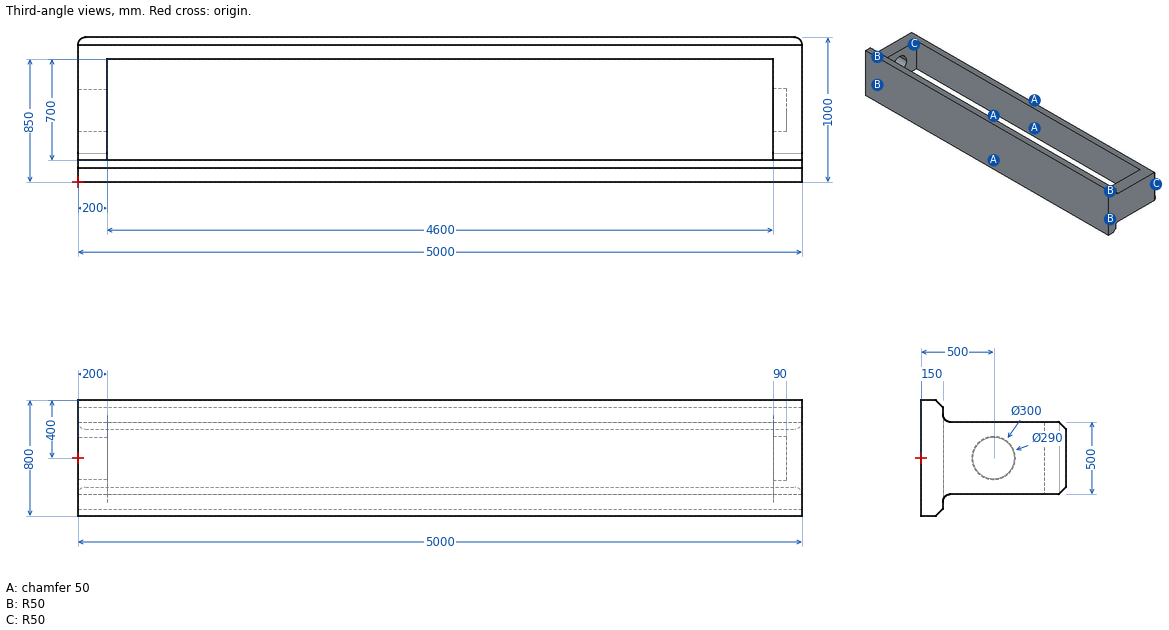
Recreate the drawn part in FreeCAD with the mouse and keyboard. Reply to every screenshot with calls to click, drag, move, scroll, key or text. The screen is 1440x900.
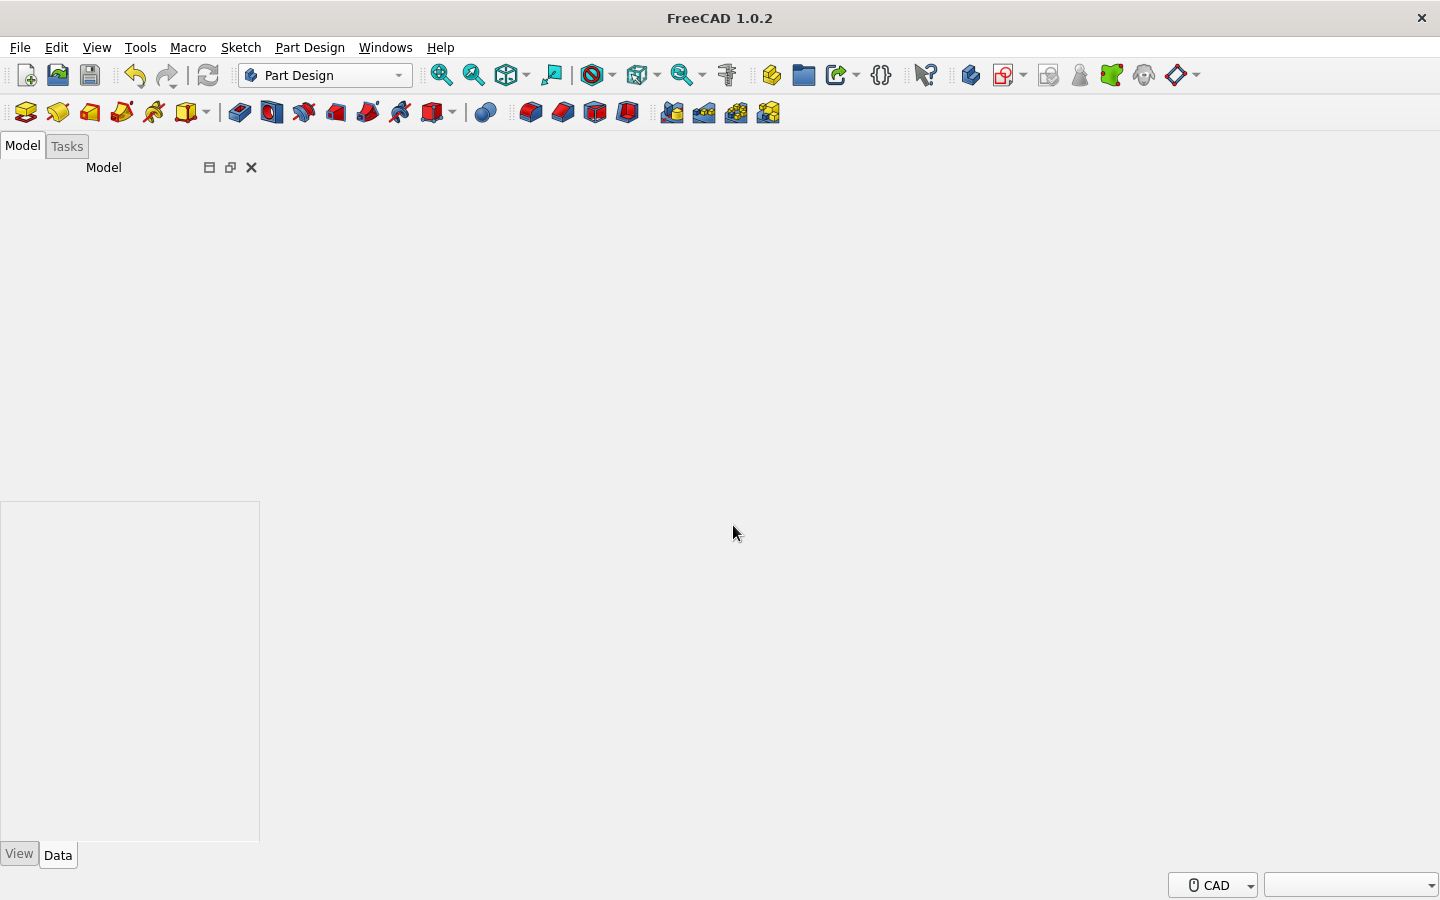
key(ctrl+n)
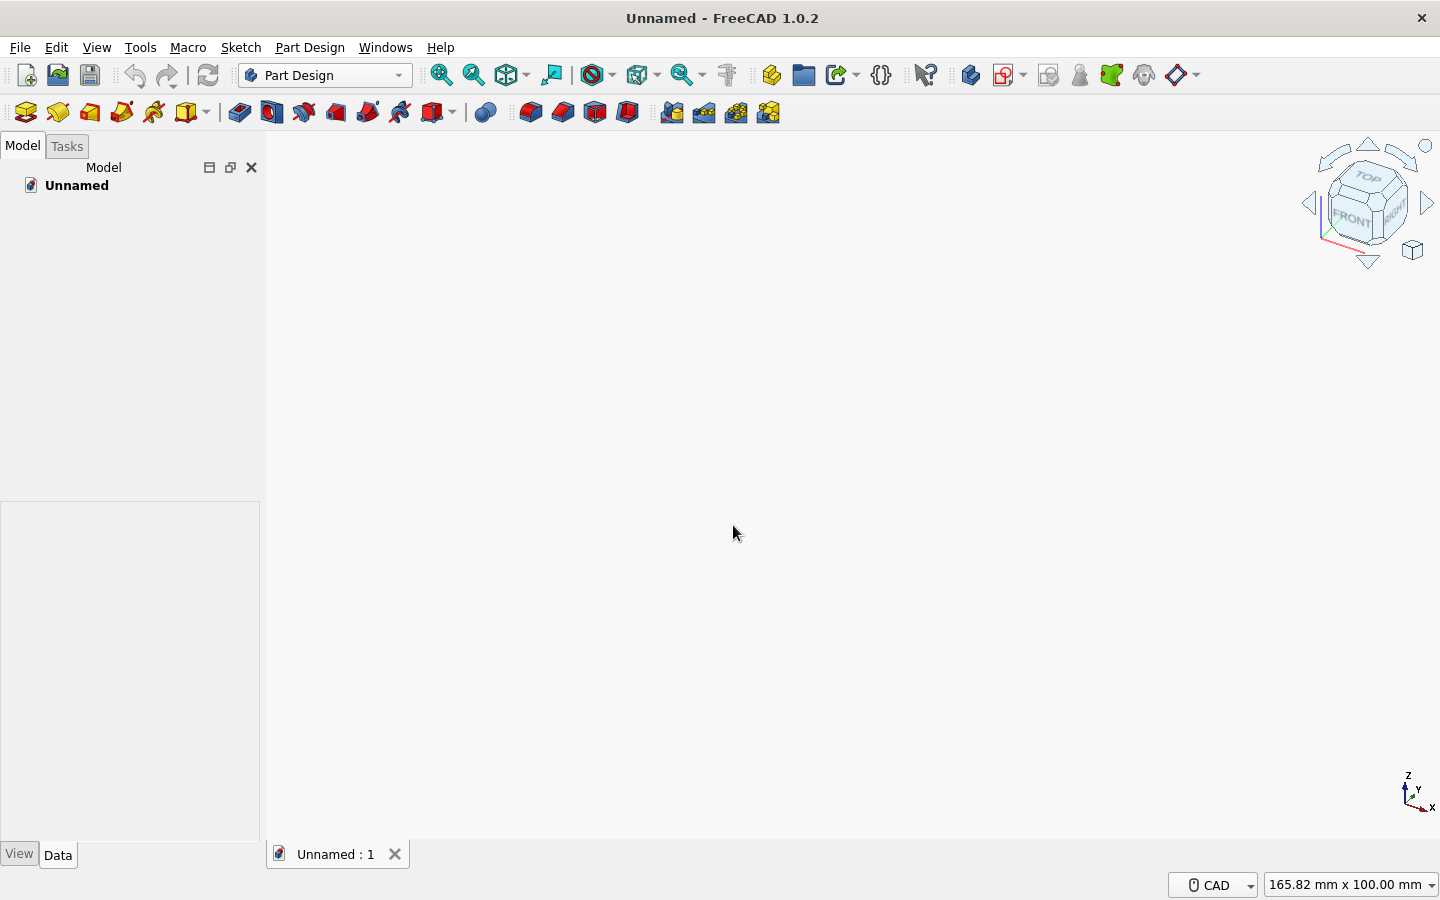
click(1004, 76)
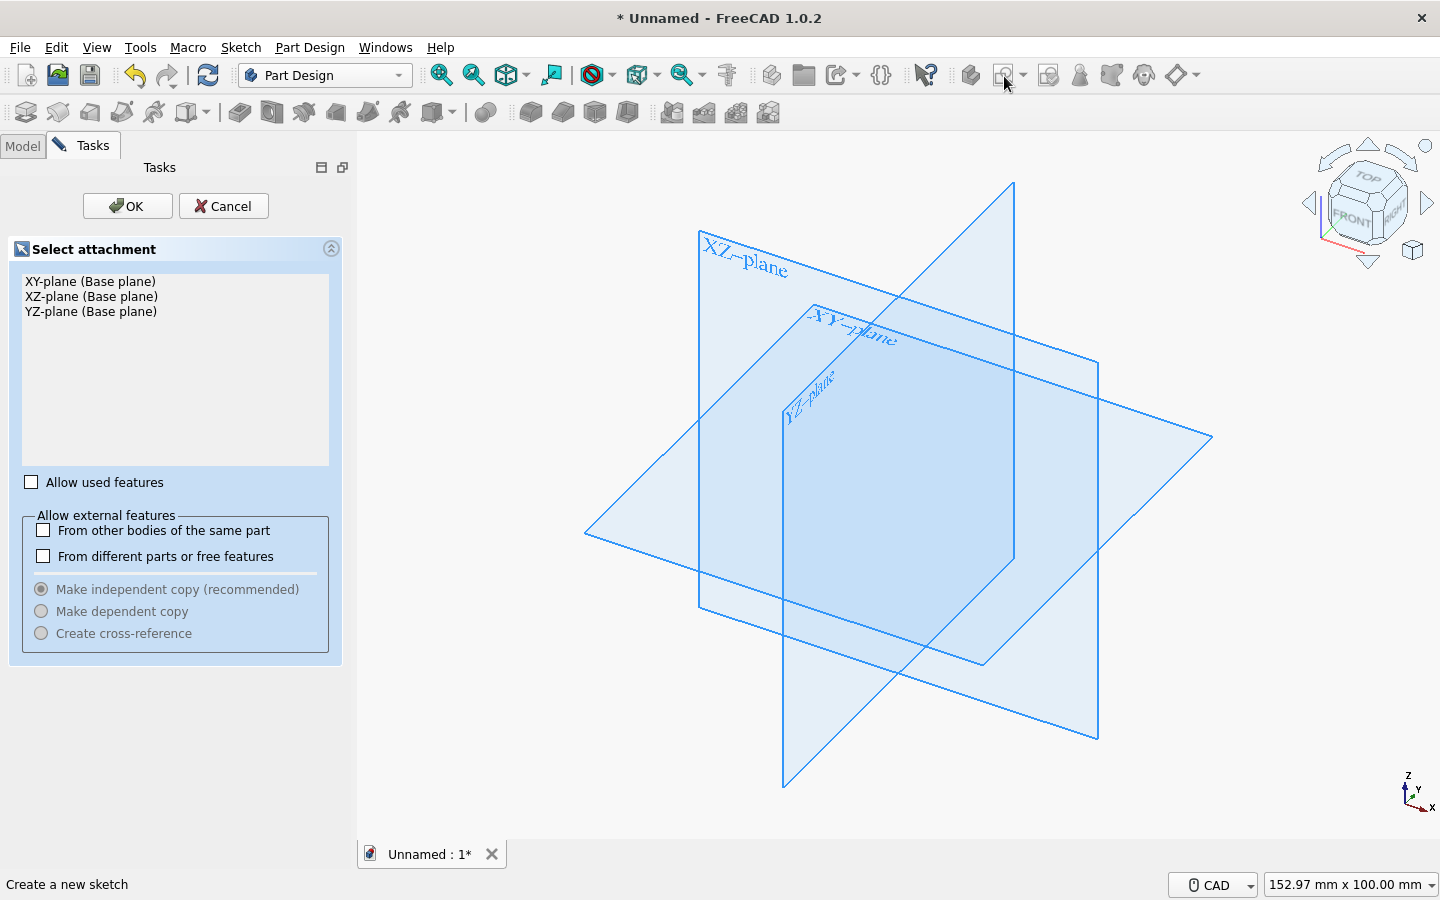
click(82, 282)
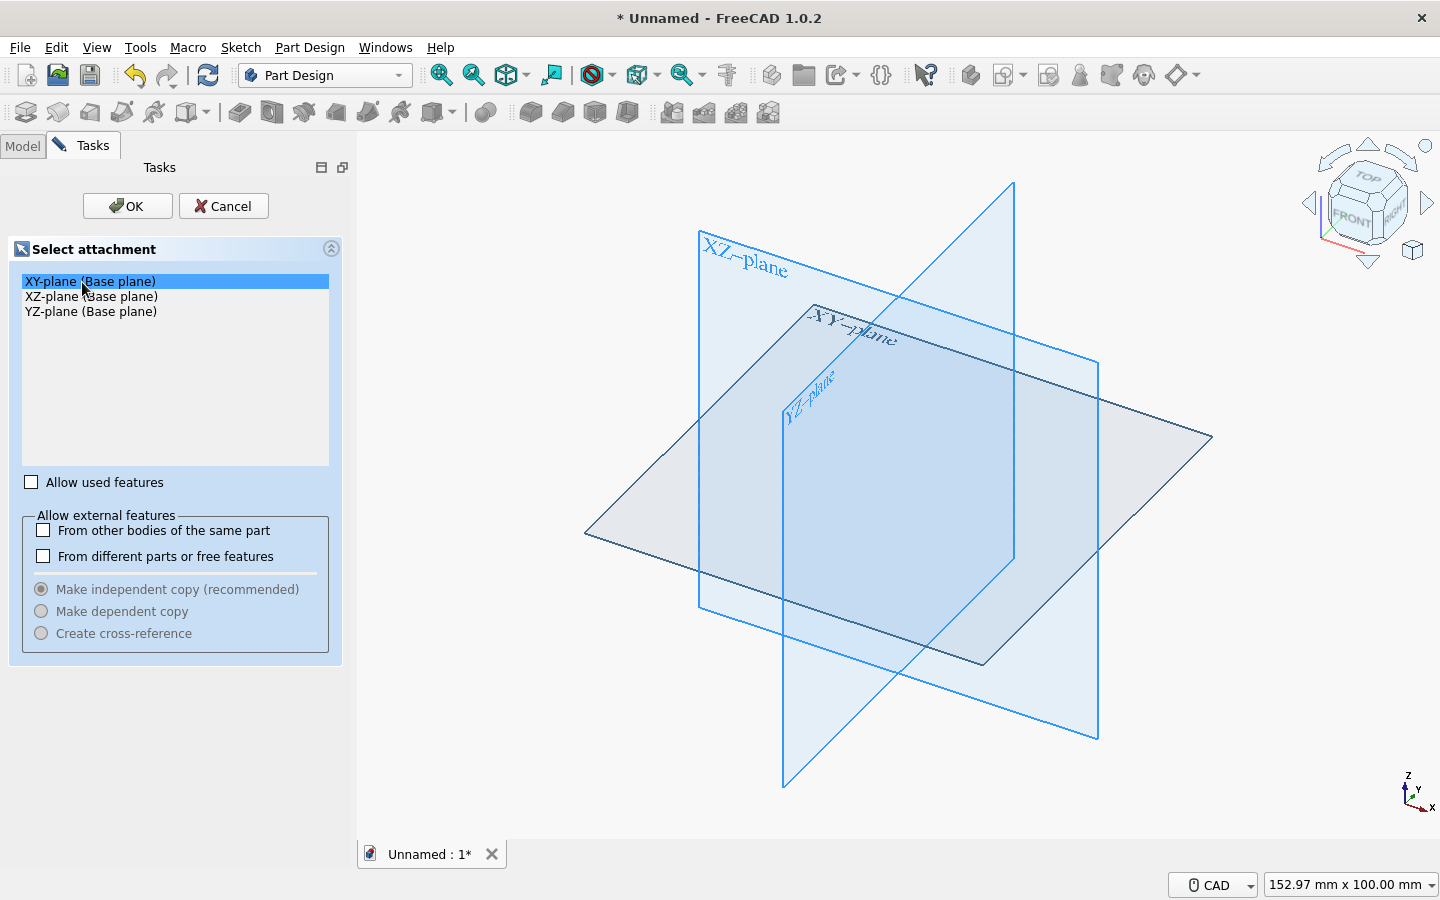
click(128, 206)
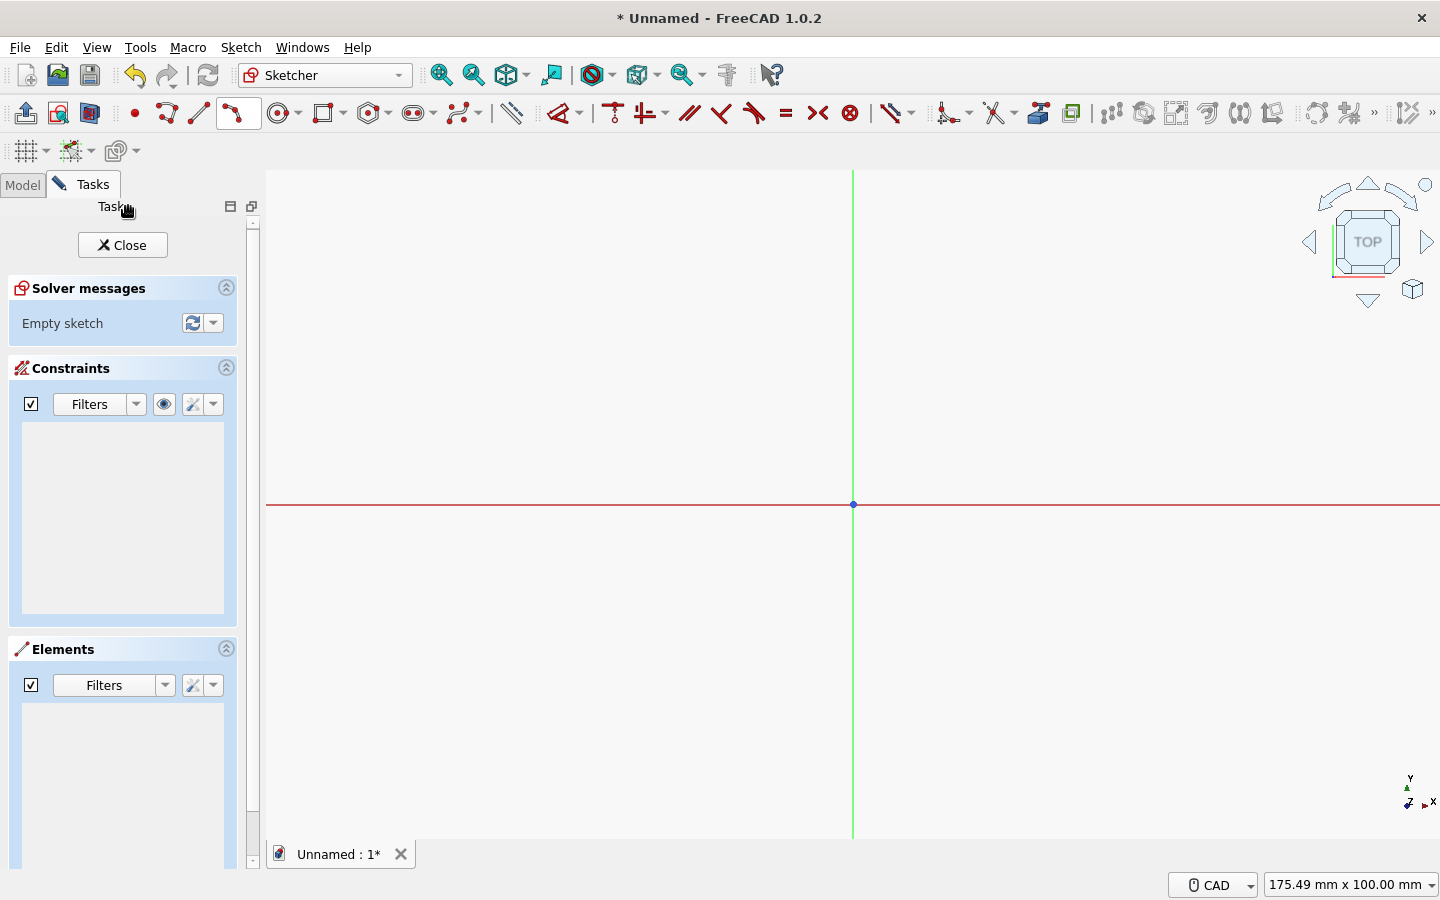
scroll(313, 598, down, 18)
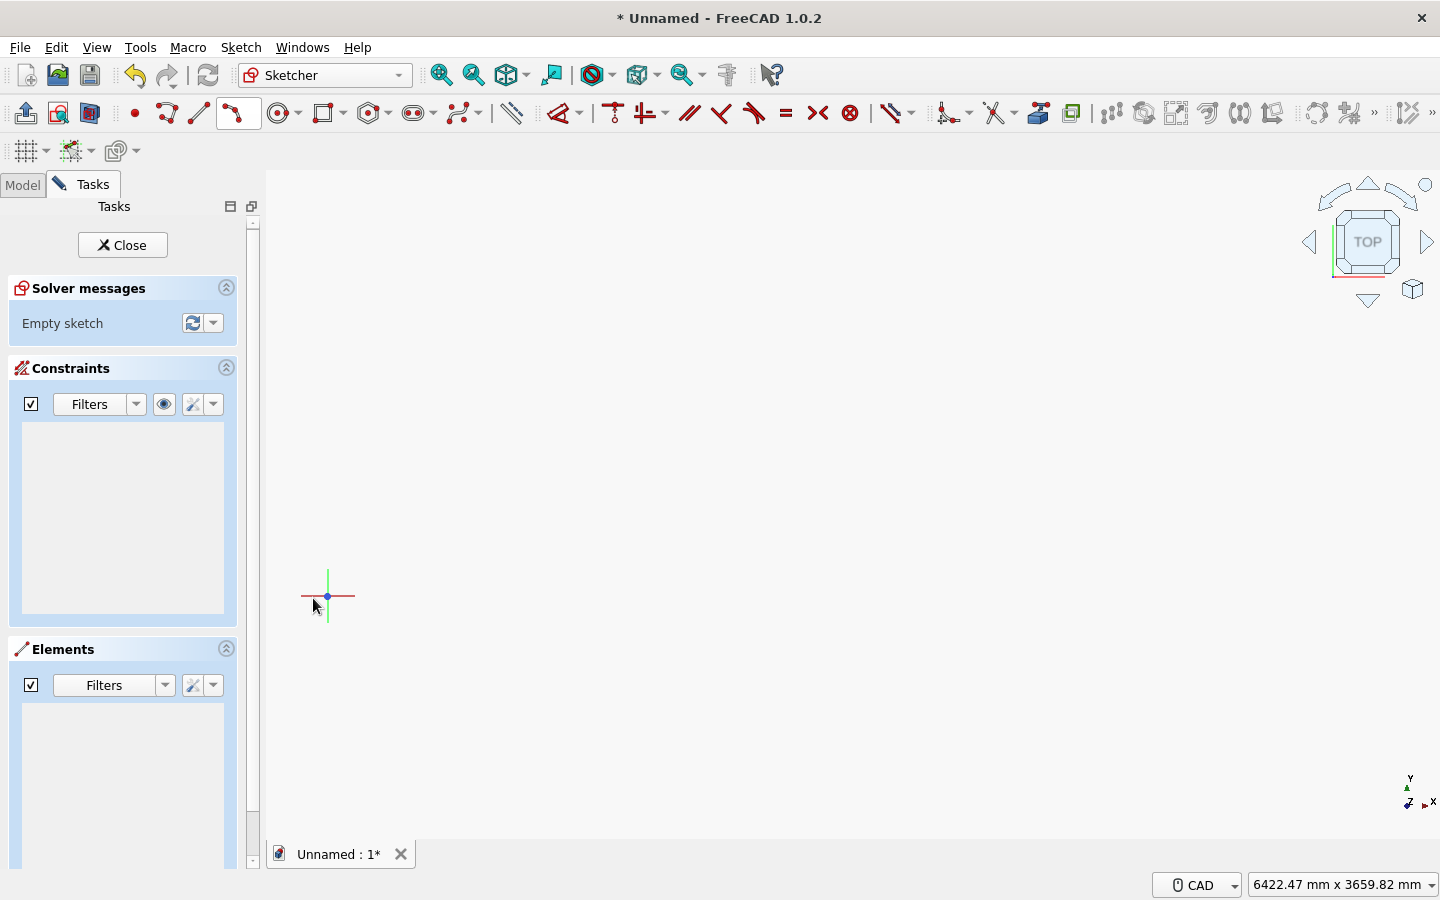
key(g)
key(r)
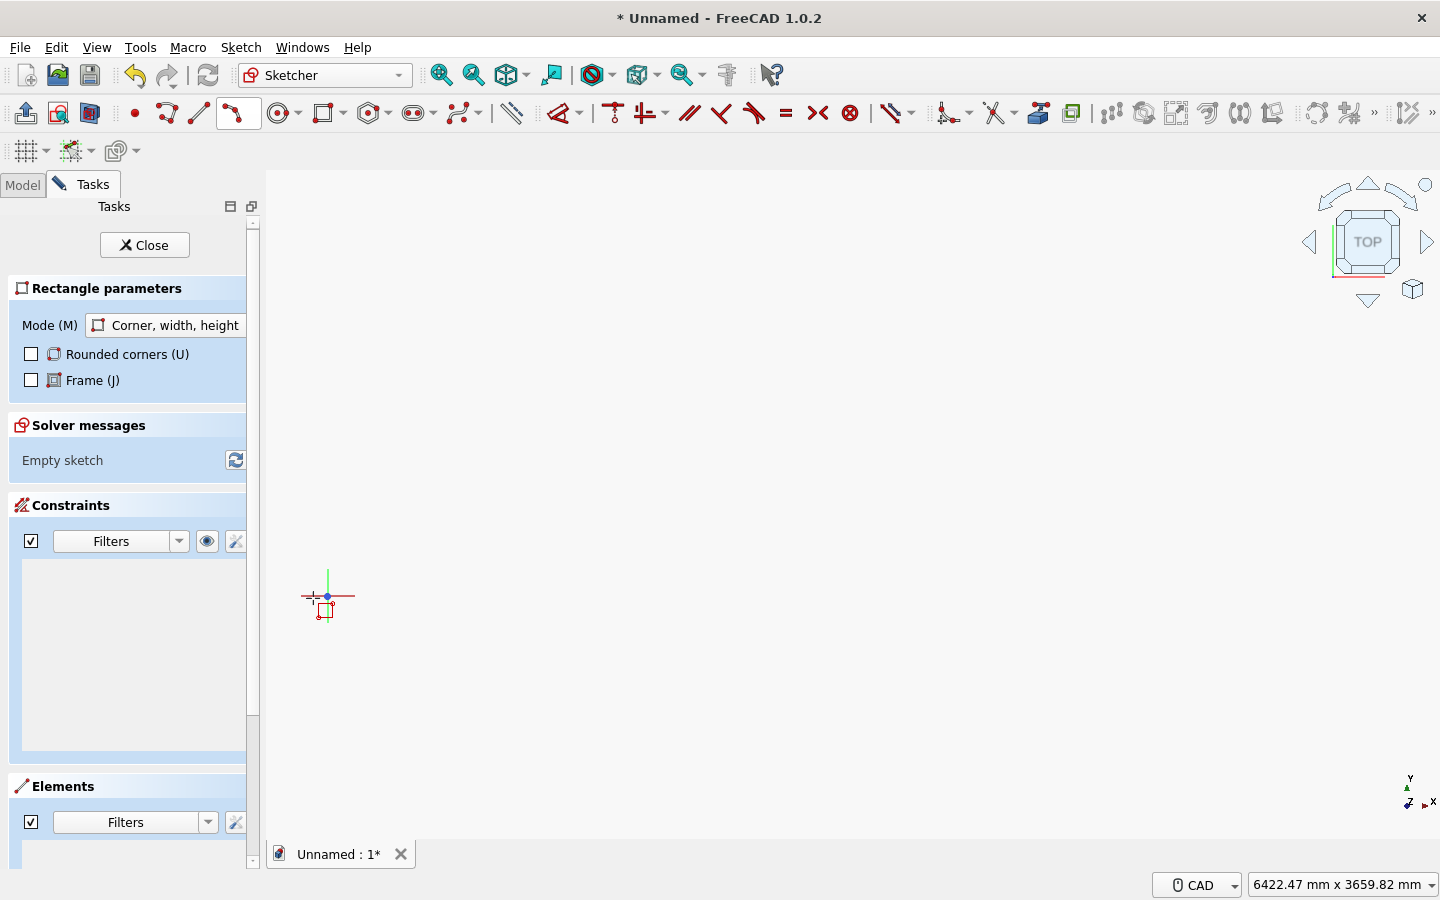
click(328, 596)
click(1242, 413)
key(Escape)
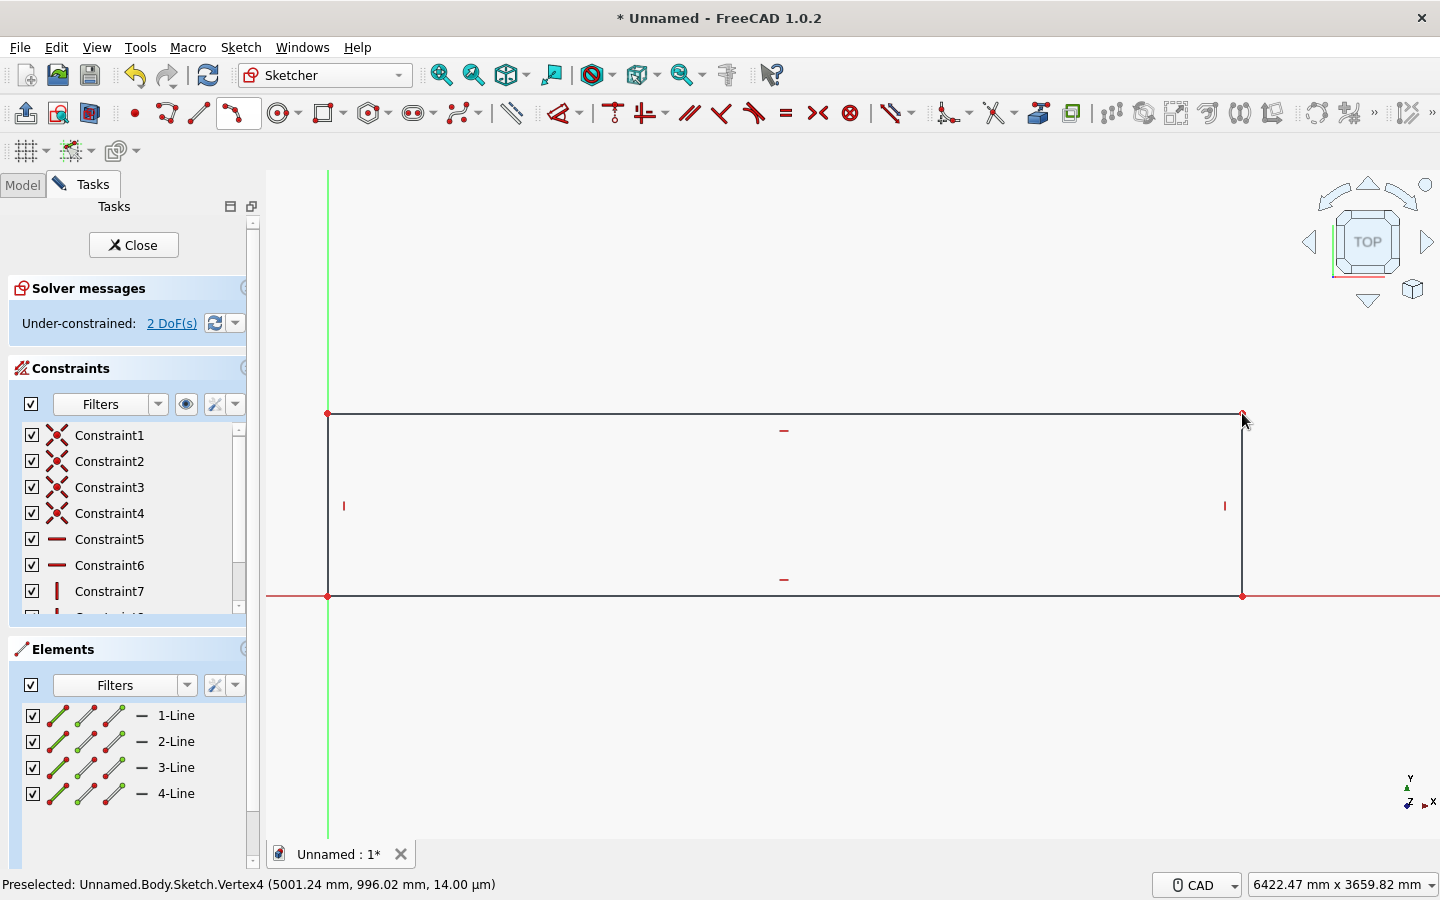
click(558, 114)